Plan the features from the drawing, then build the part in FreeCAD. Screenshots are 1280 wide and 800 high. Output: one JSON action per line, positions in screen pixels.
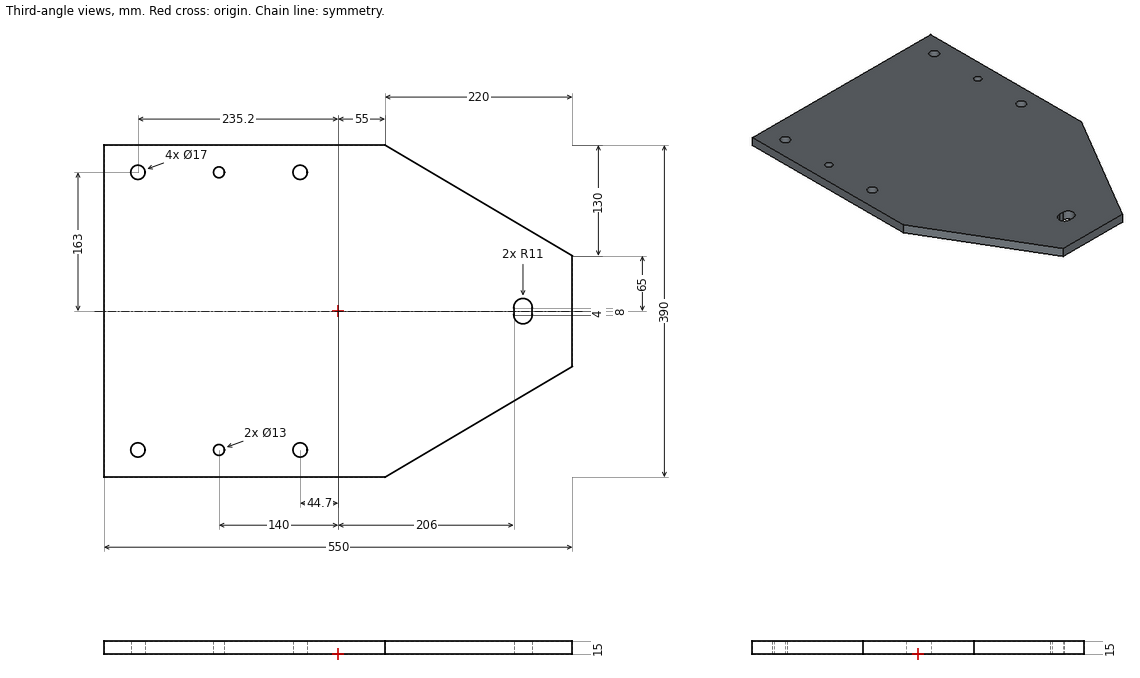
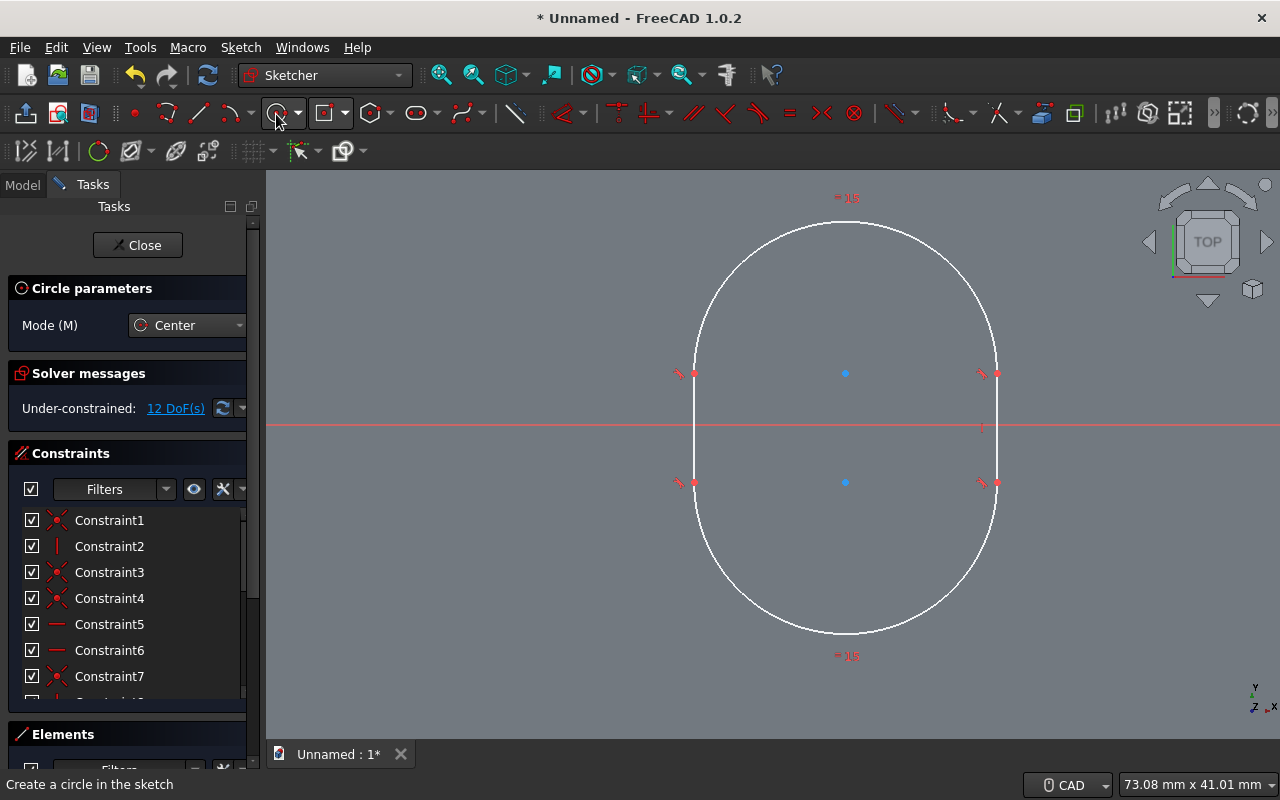
{"action": "scroll", "coordinate": [876, 456], "scroll_direction": "down", "scroll_amount": 14}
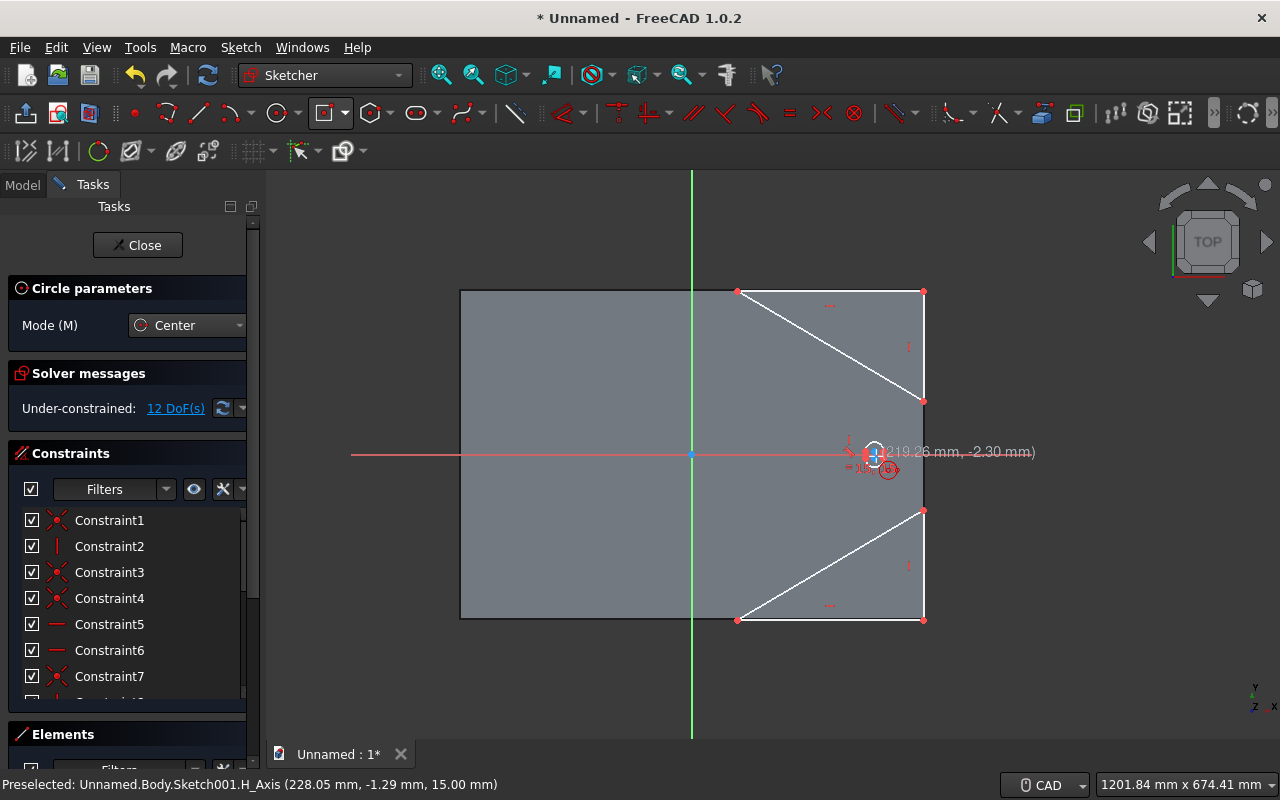
{"action": "scroll", "coordinate": [493, 317], "scroll_direction": "up", "scroll_amount": 6}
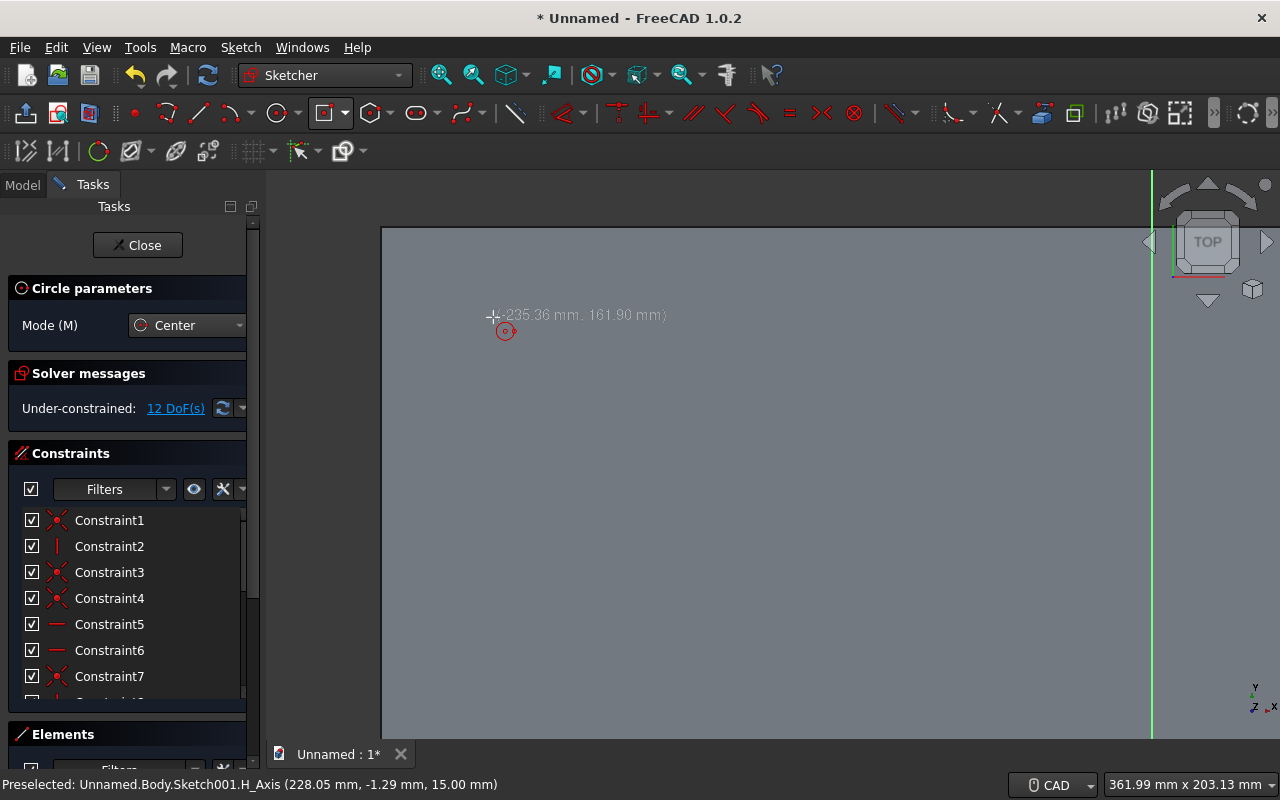
{"action": "left_click", "coordinate": [493, 317]}
{"action": "left_click", "coordinate": [510, 300]}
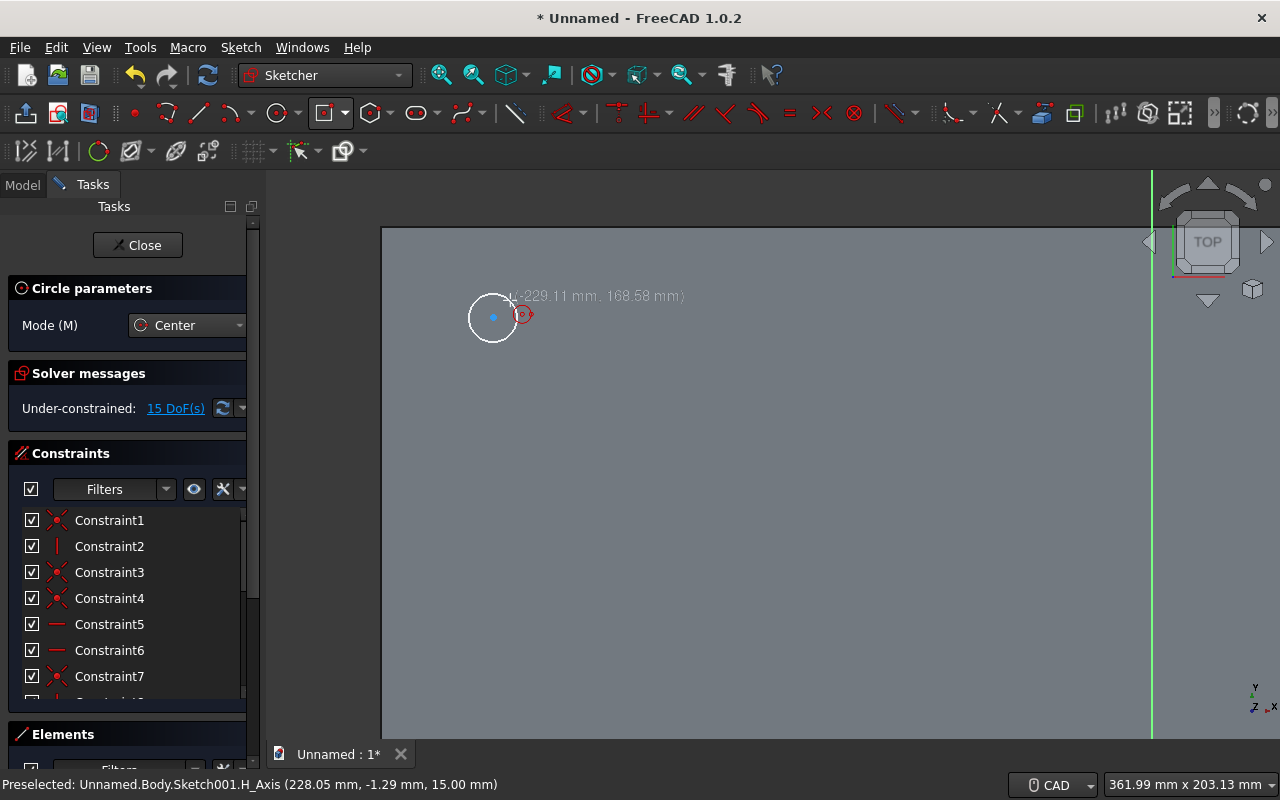
{"action": "scroll", "coordinate": [493, 317], "scroll_direction": "down", "scroll_amount": 6}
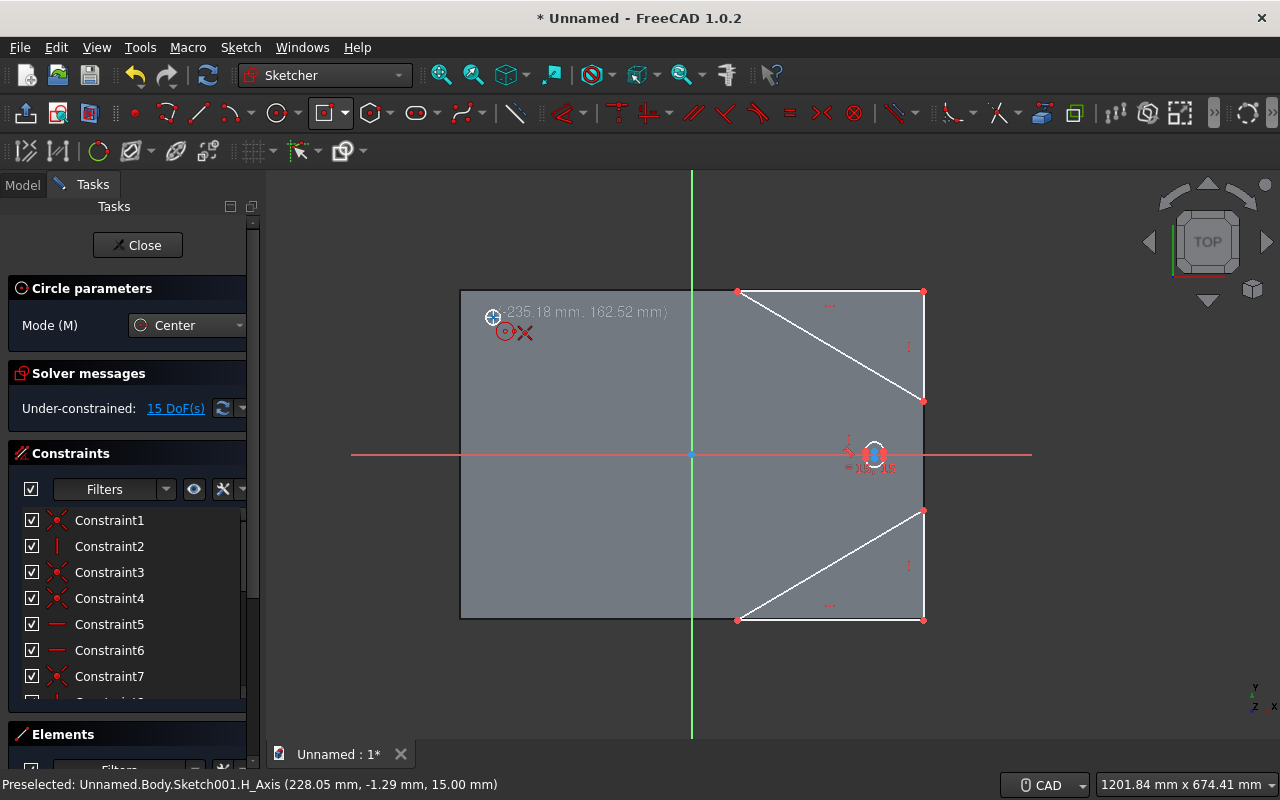
{"action": "scroll", "coordinate": [493, 592], "scroll_direction": "up", "scroll_amount": 6}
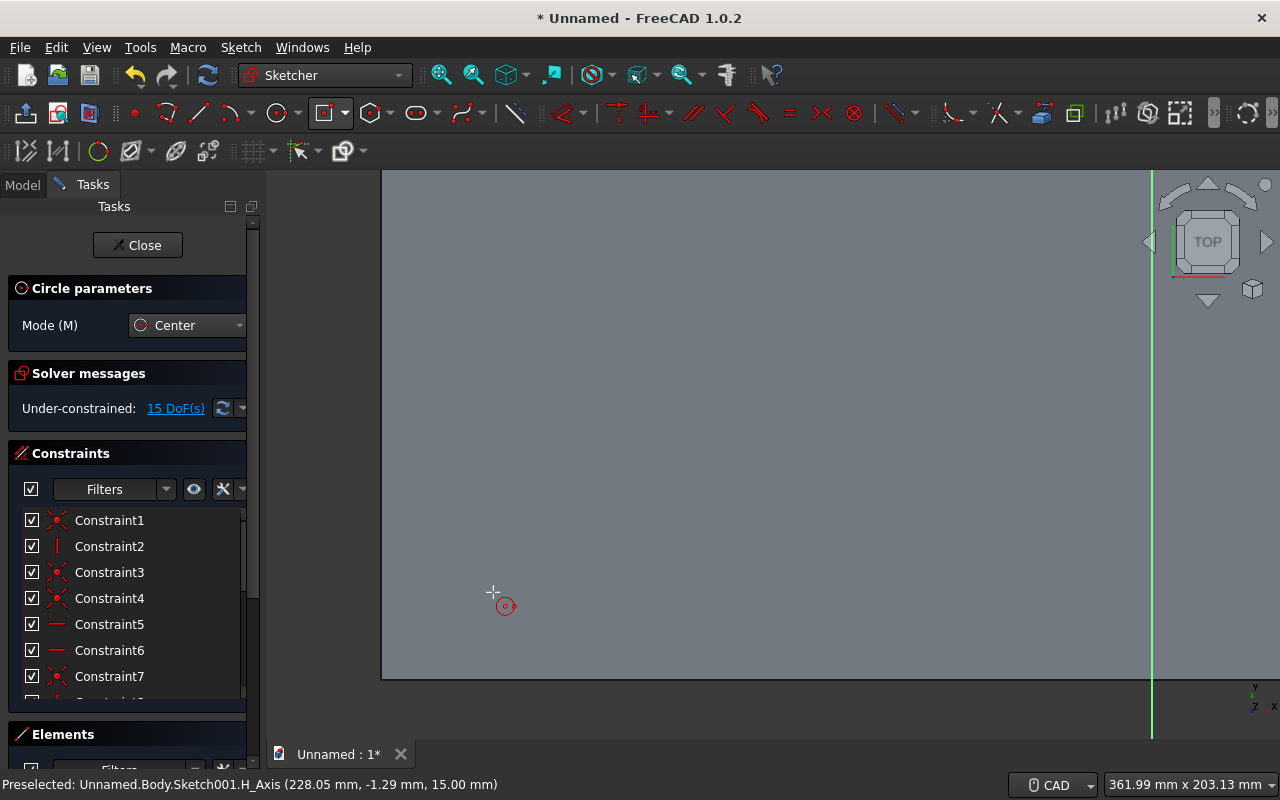
{"action": "left_click", "coordinate": [493, 591]}
{"action": "left_click", "coordinate": [510, 574]}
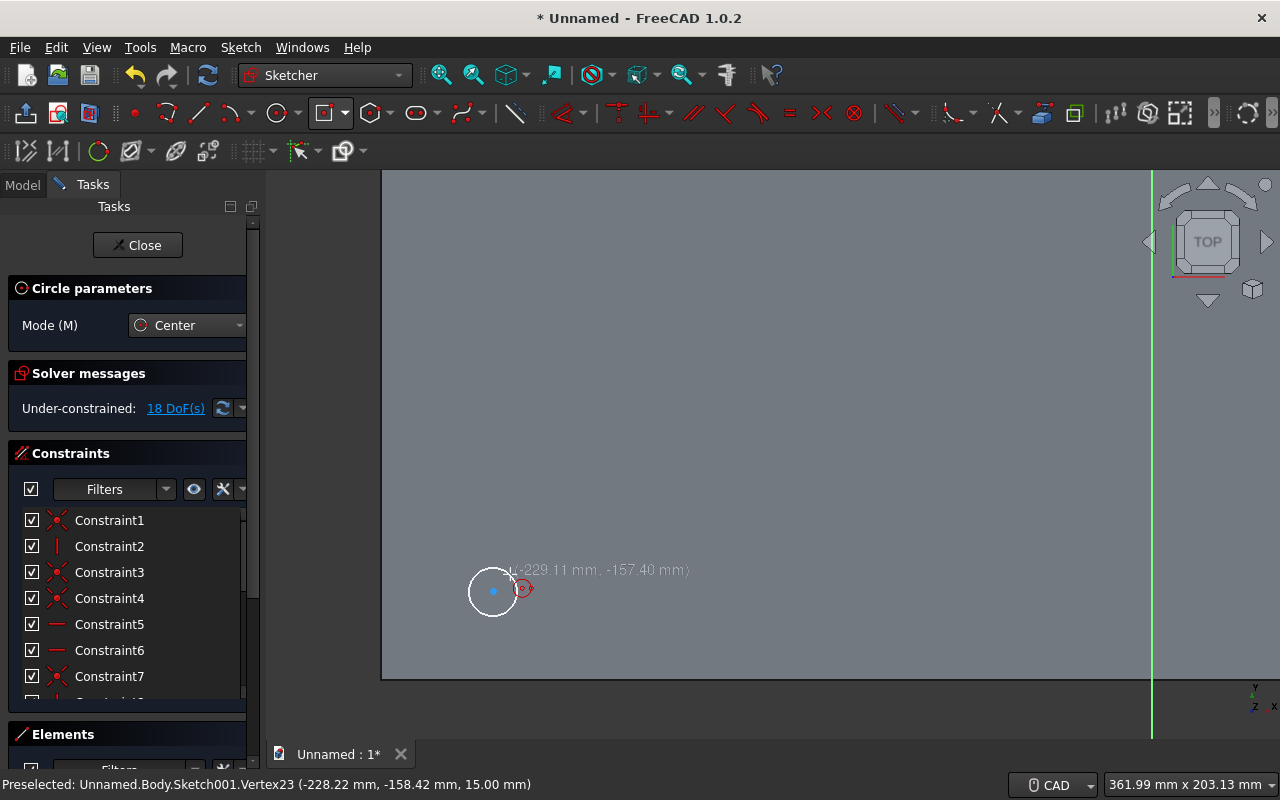
{"action": "scroll", "coordinate": [760, 591], "scroll_direction": "up", "scroll_amount": 2}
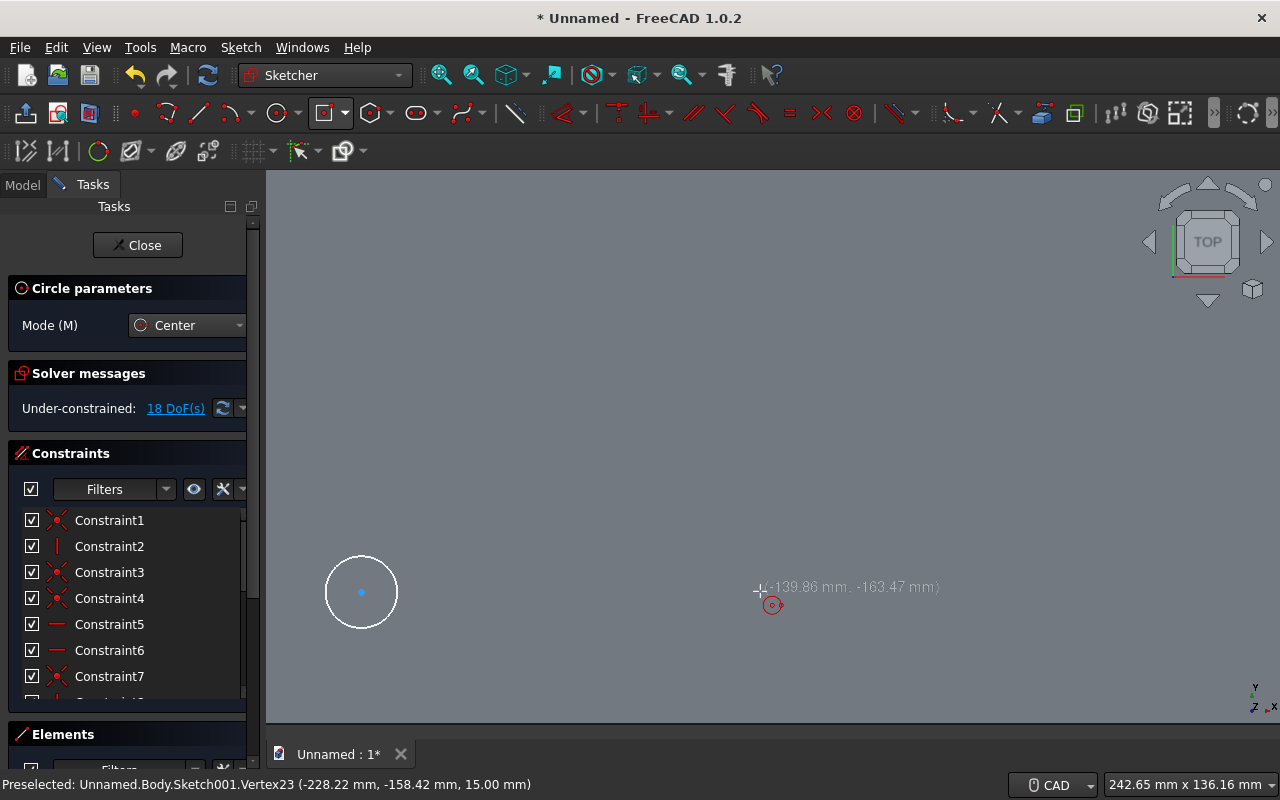
{"action": "scroll", "coordinate": [526, 592], "scroll_direction": "down", "scroll_amount": 8}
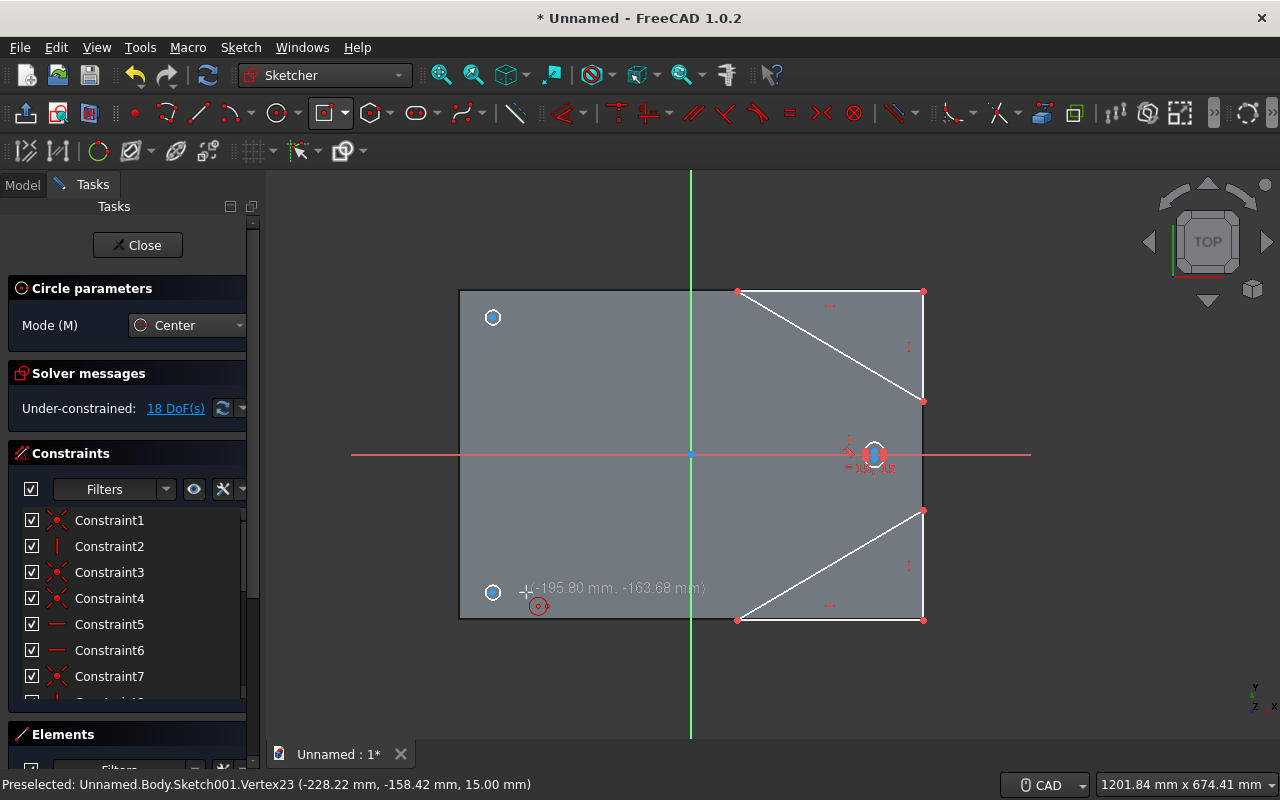
{"action": "left_click", "coordinate": [573, 592]}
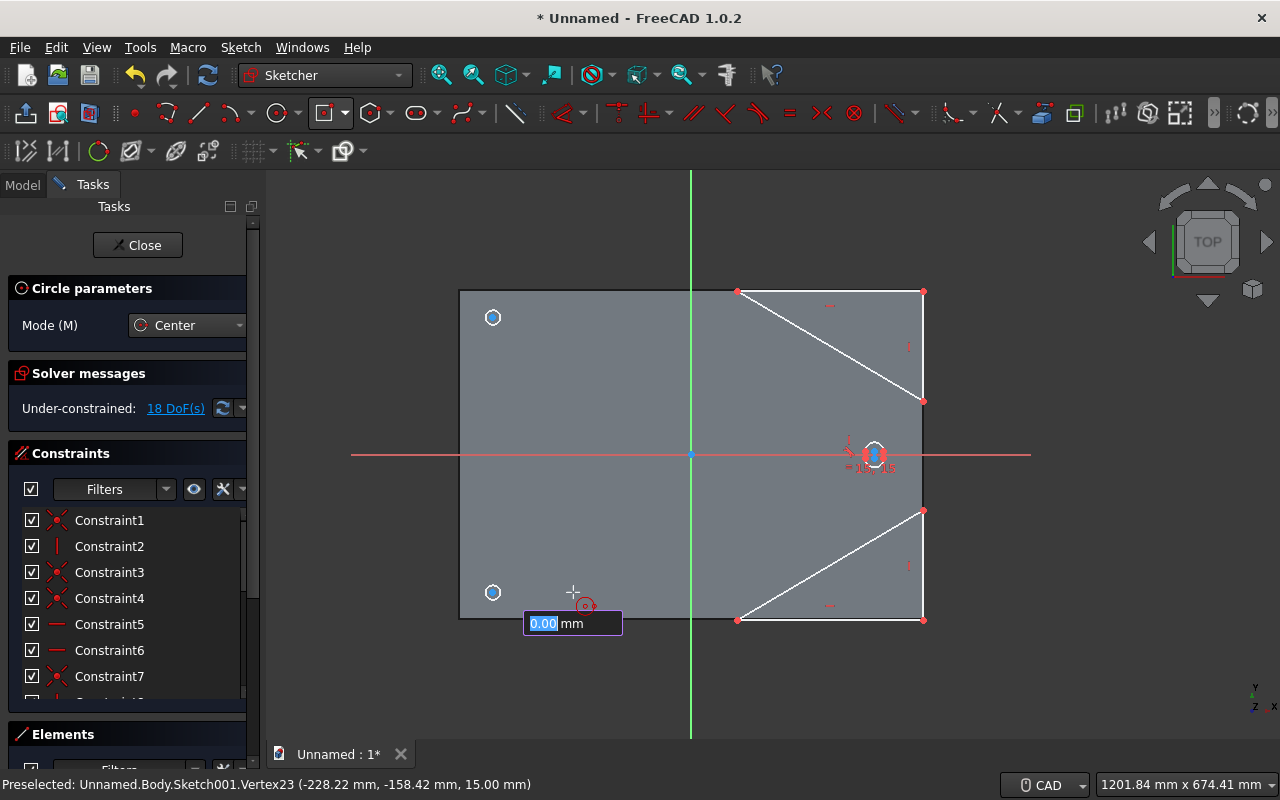
{"action": "scroll", "coordinate": [577, 588], "scroll_direction": "up", "scroll_amount": 6}